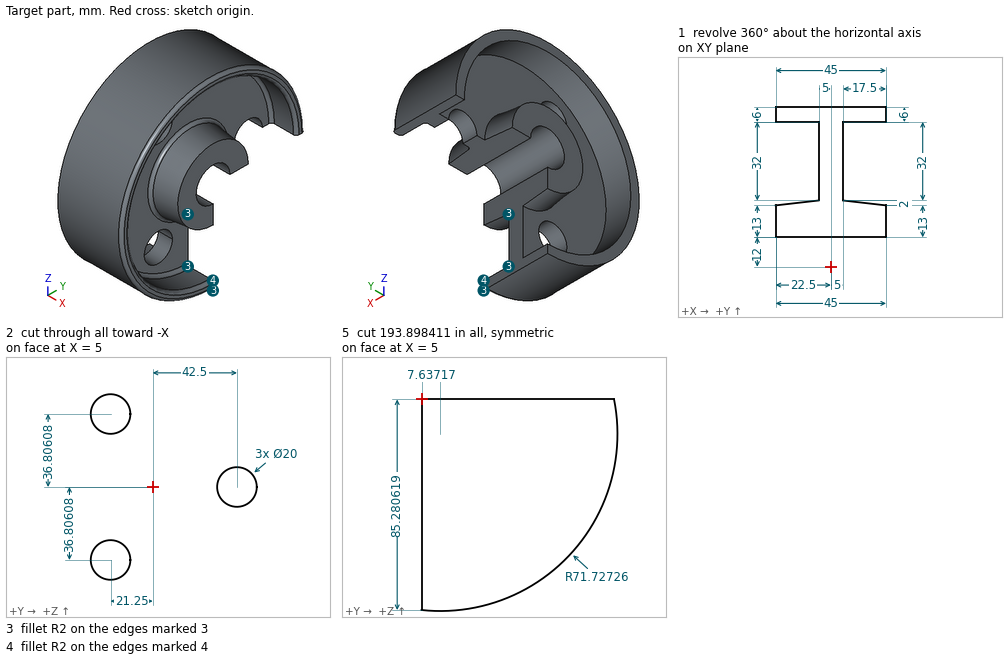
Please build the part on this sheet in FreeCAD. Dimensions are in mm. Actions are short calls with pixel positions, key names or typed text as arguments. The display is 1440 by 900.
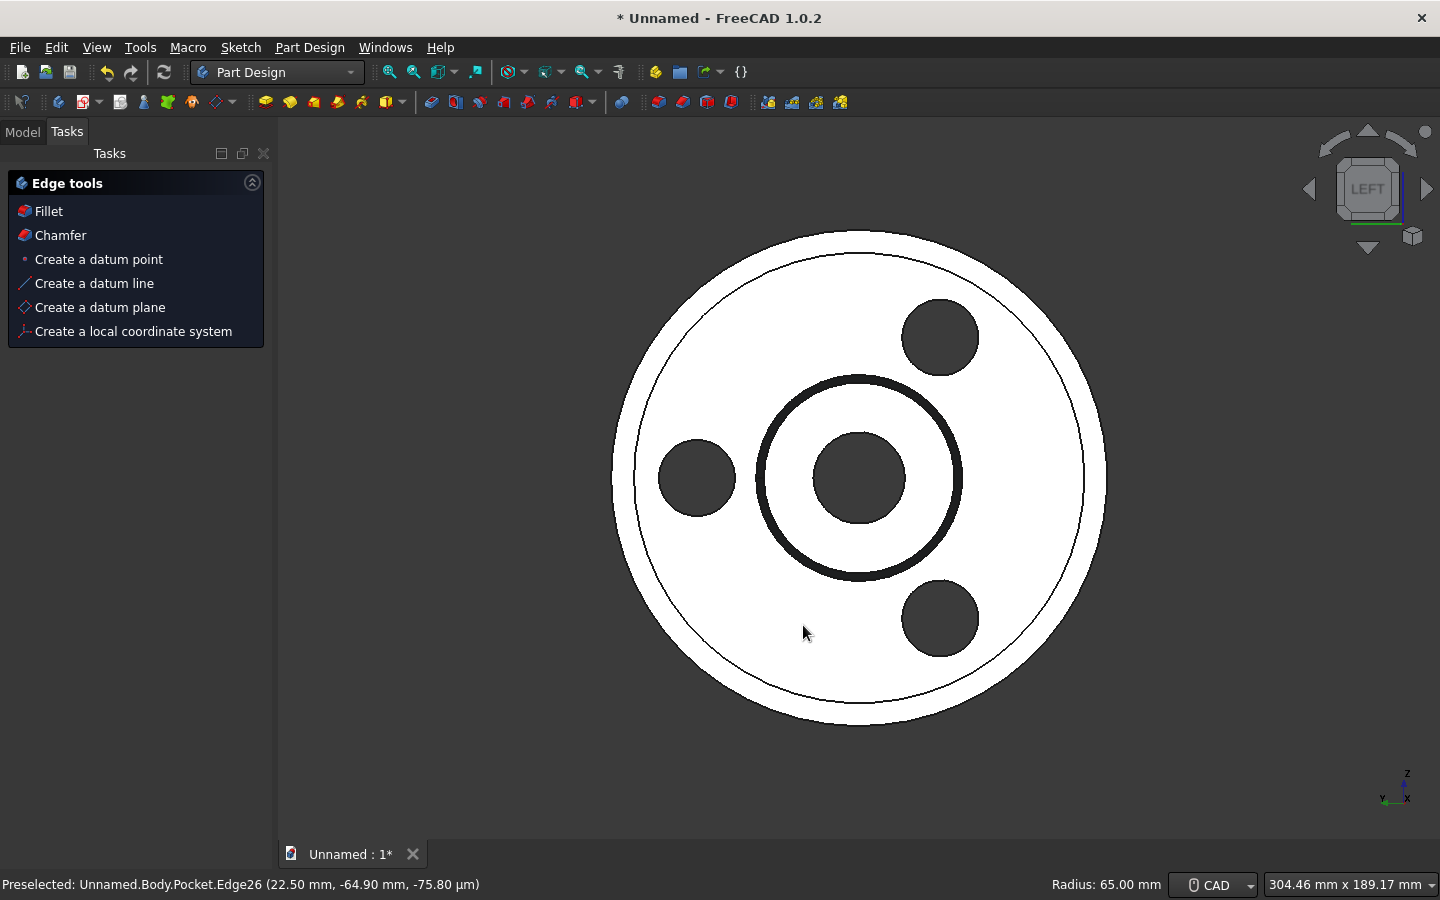
key(v)
key(3)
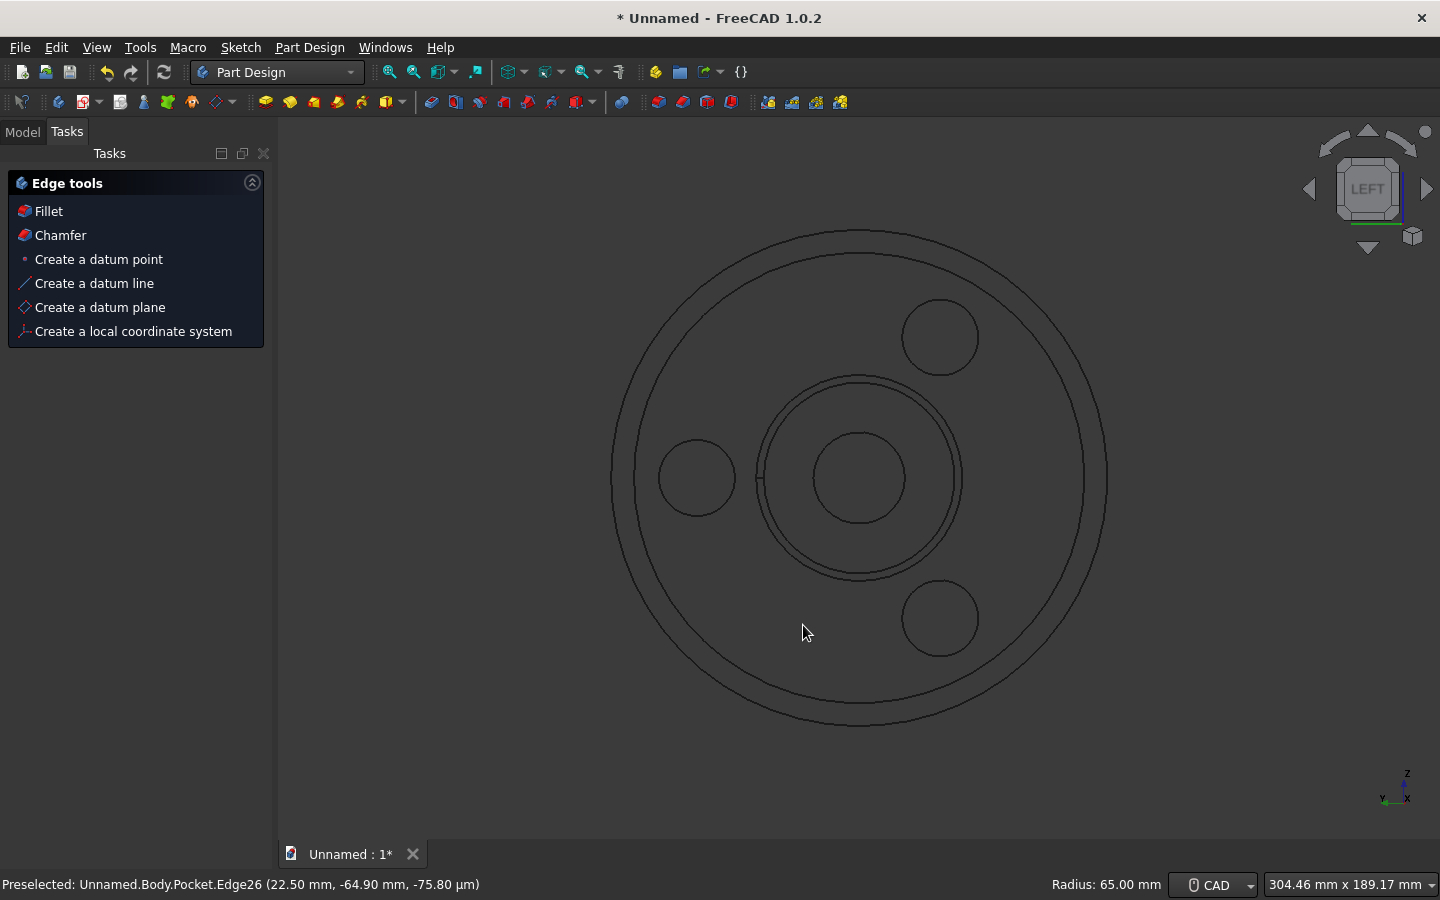
key(0)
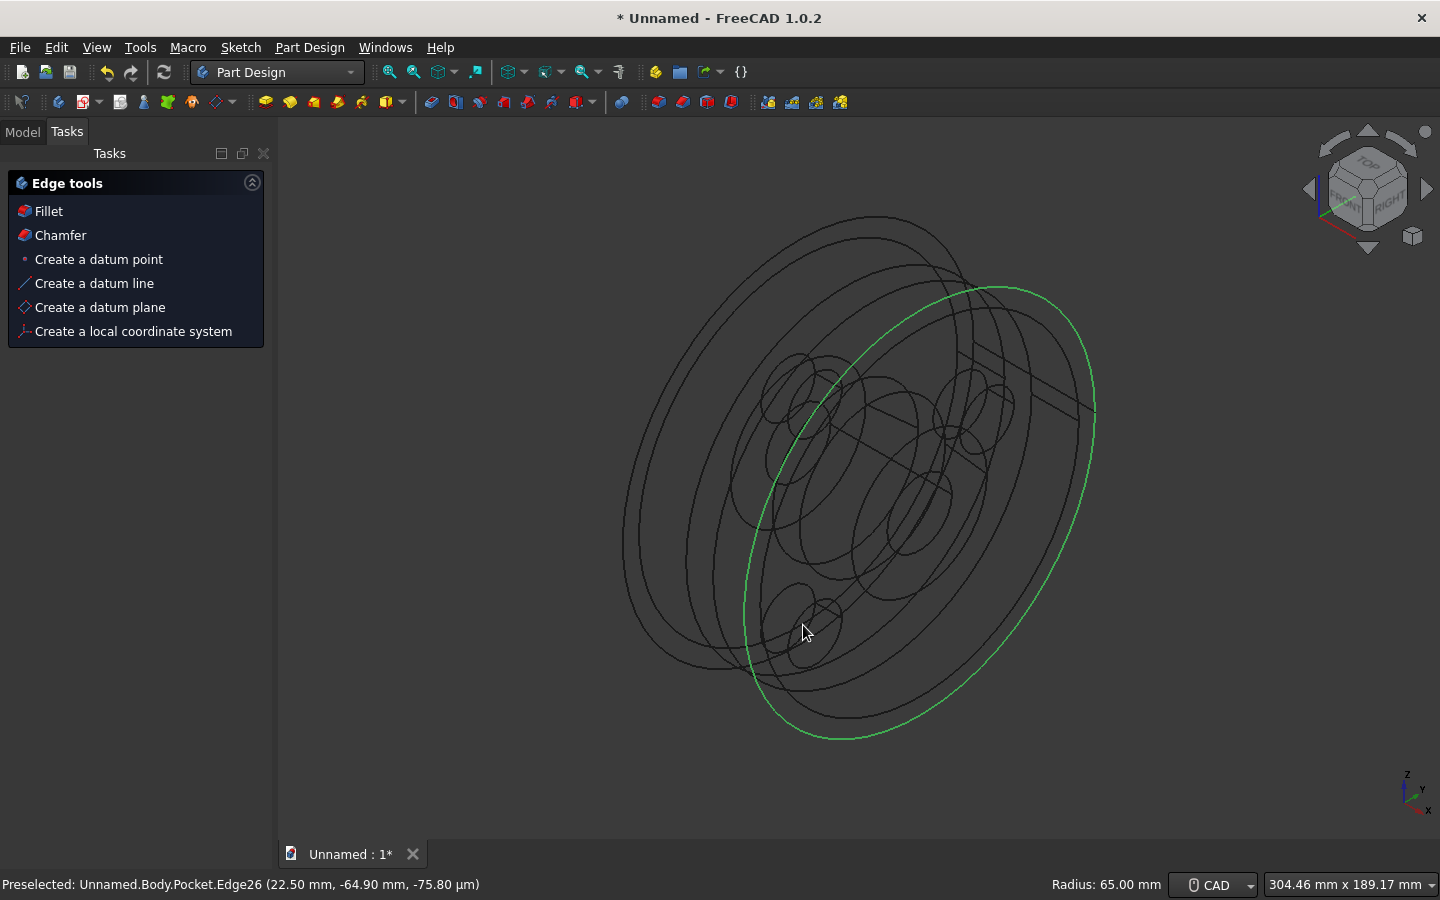
click(713, 577, ctrl)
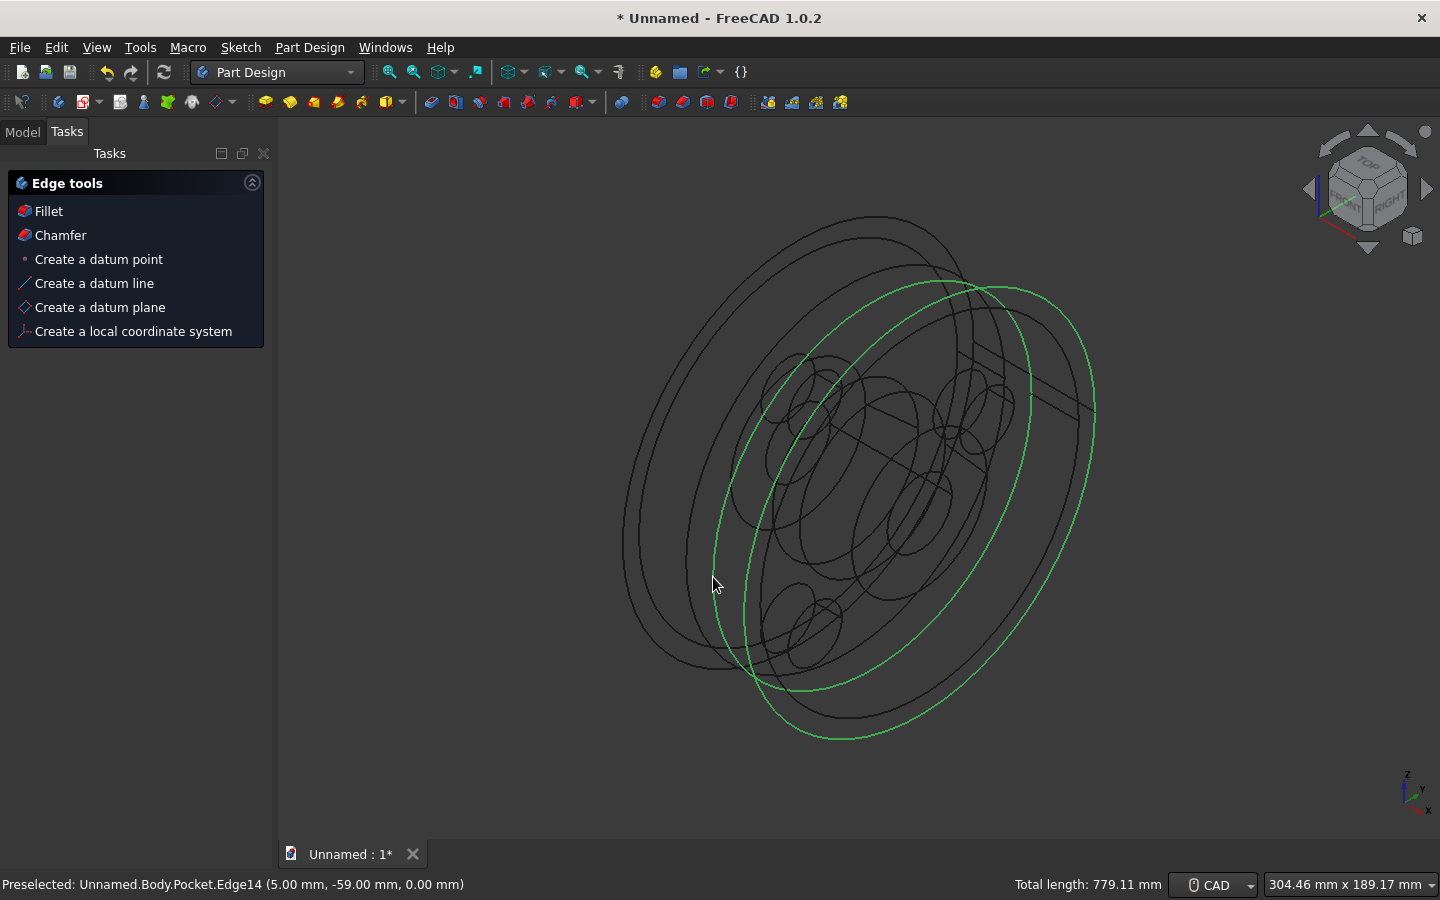
click(799, 527, ctrl)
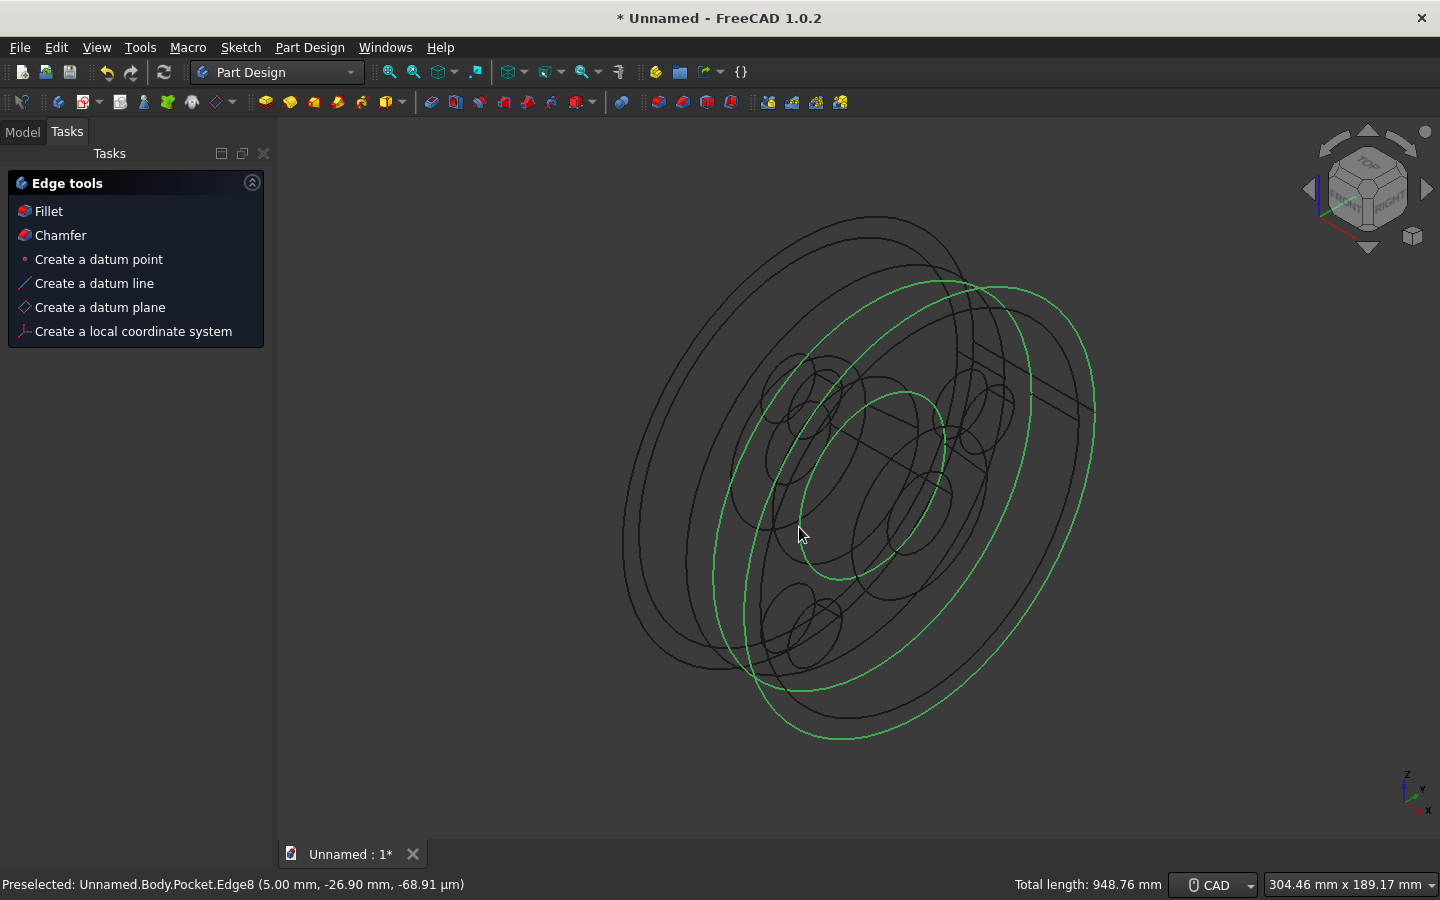
key(v)
key(1)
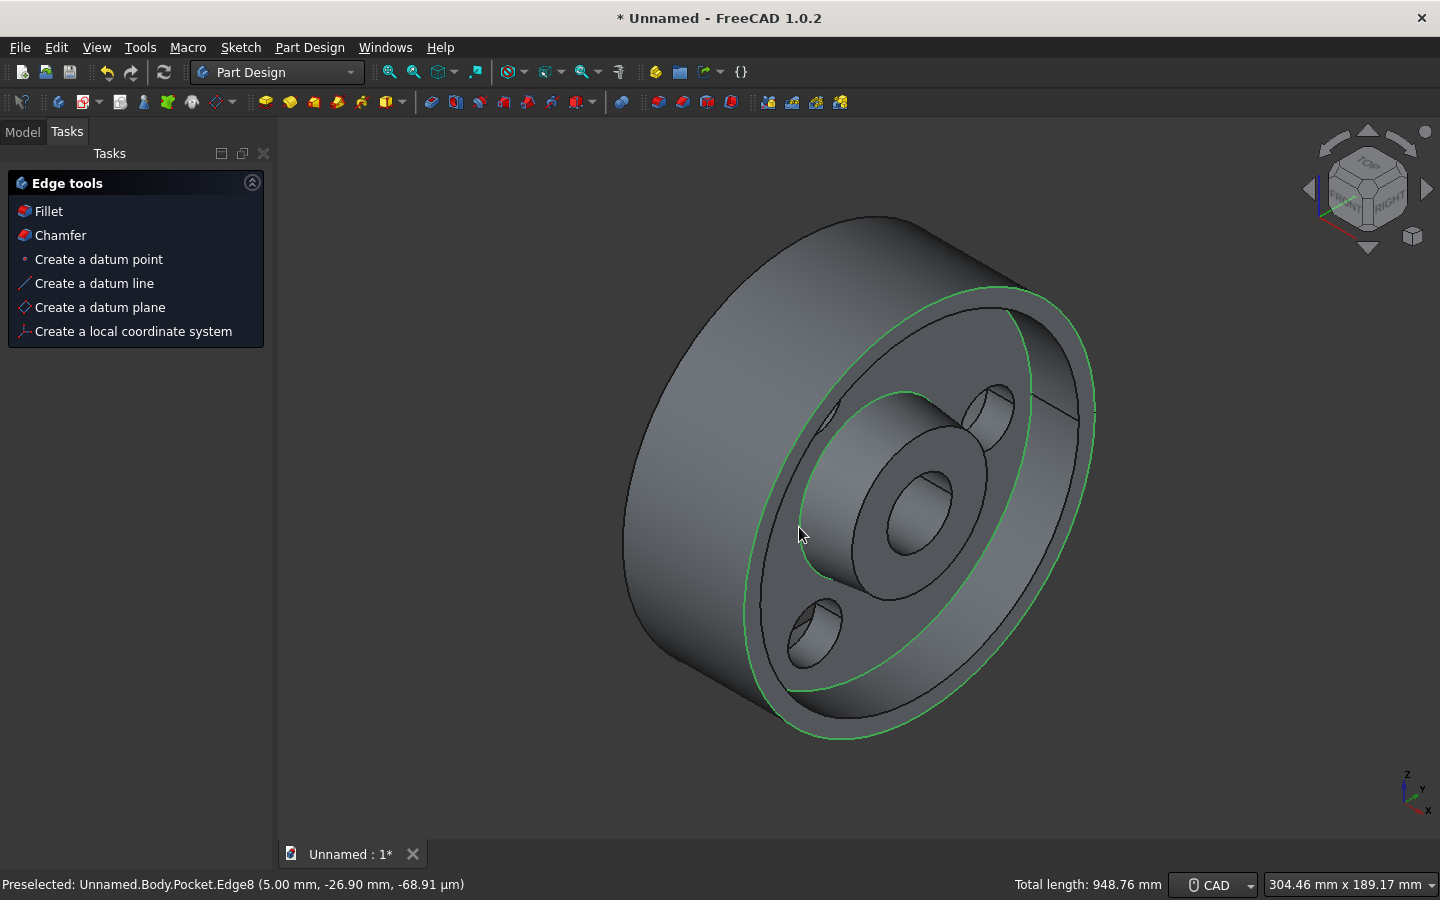
click(660, 102)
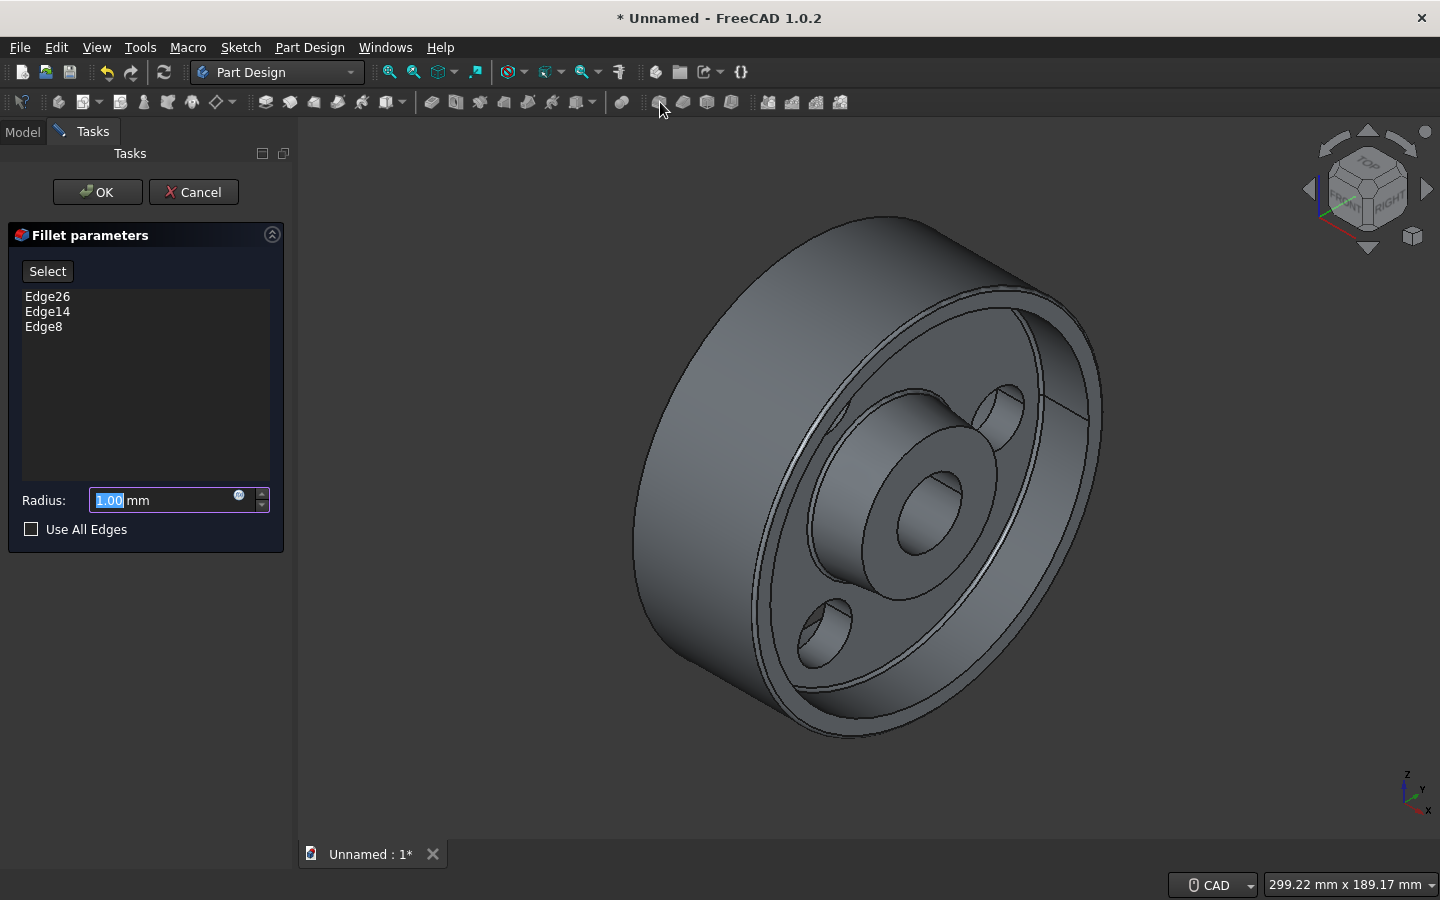
text(2)
key(Tab)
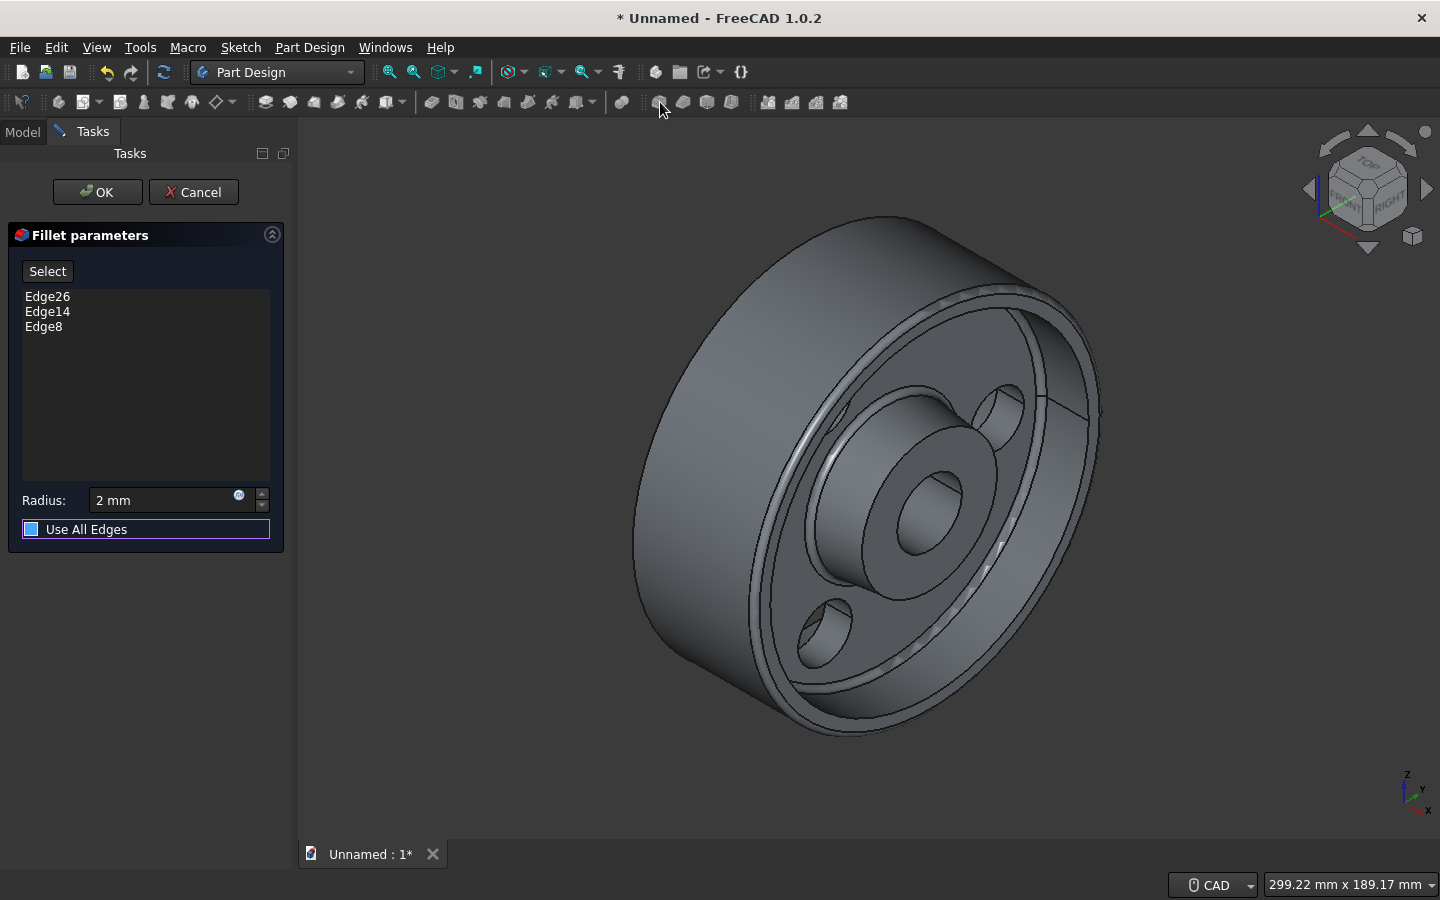
click(98, 192)